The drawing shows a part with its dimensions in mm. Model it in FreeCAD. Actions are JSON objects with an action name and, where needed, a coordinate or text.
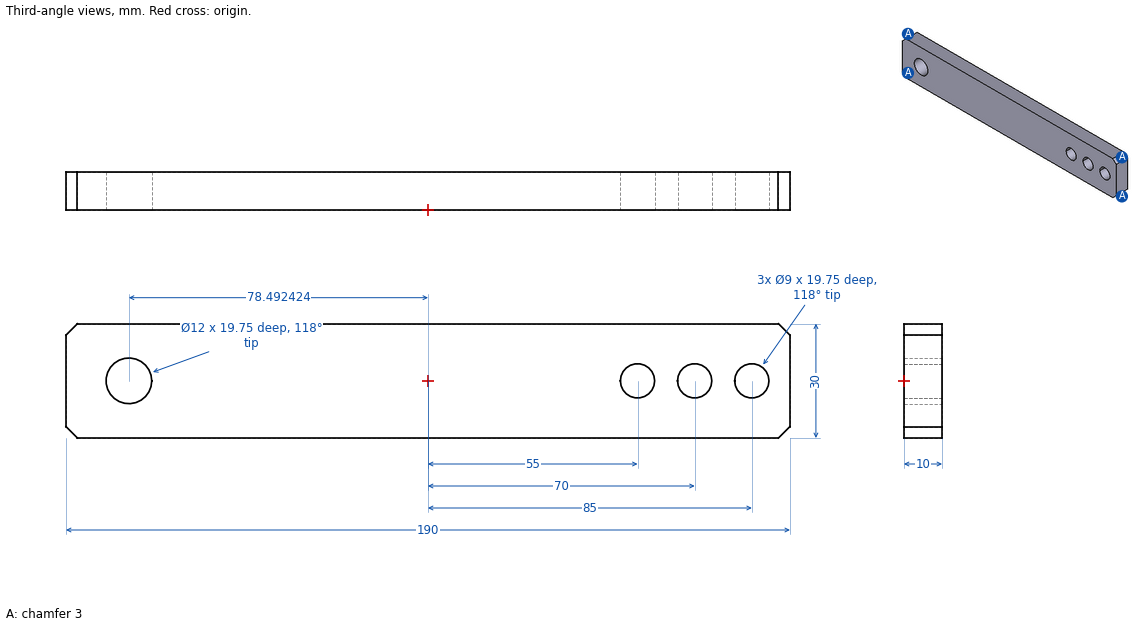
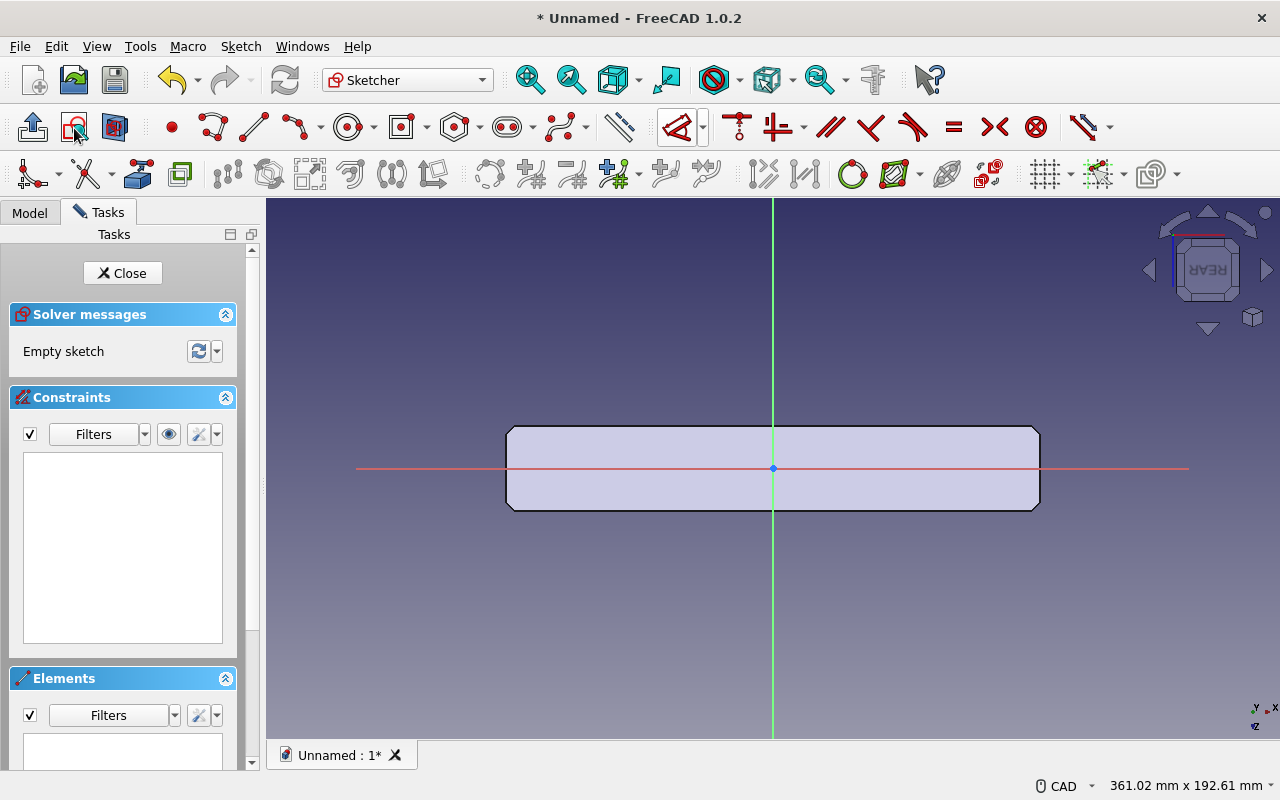
{"action": "scroll", "coordinate": [1057, 468], "scroll_direction": "up", "scroll_amount": 4}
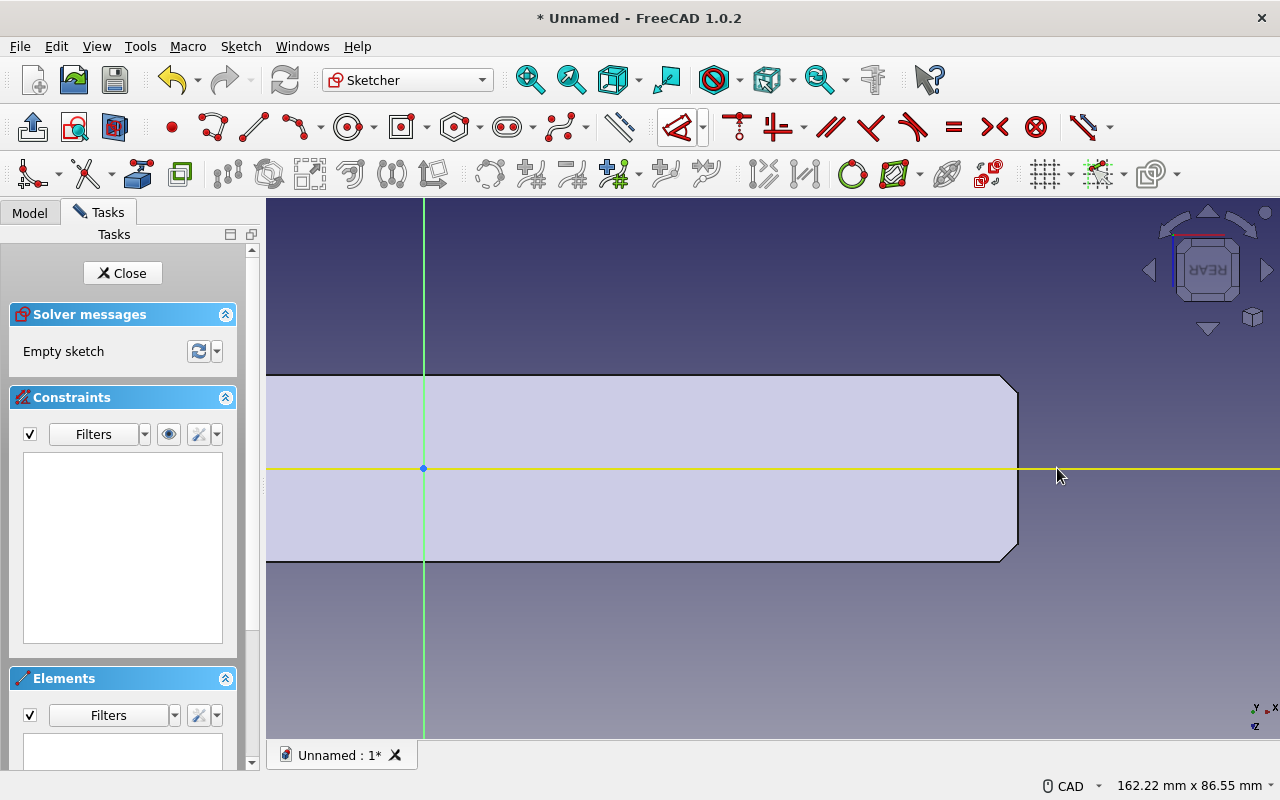
{"action": "left_click", "coordinate": [348, 128]}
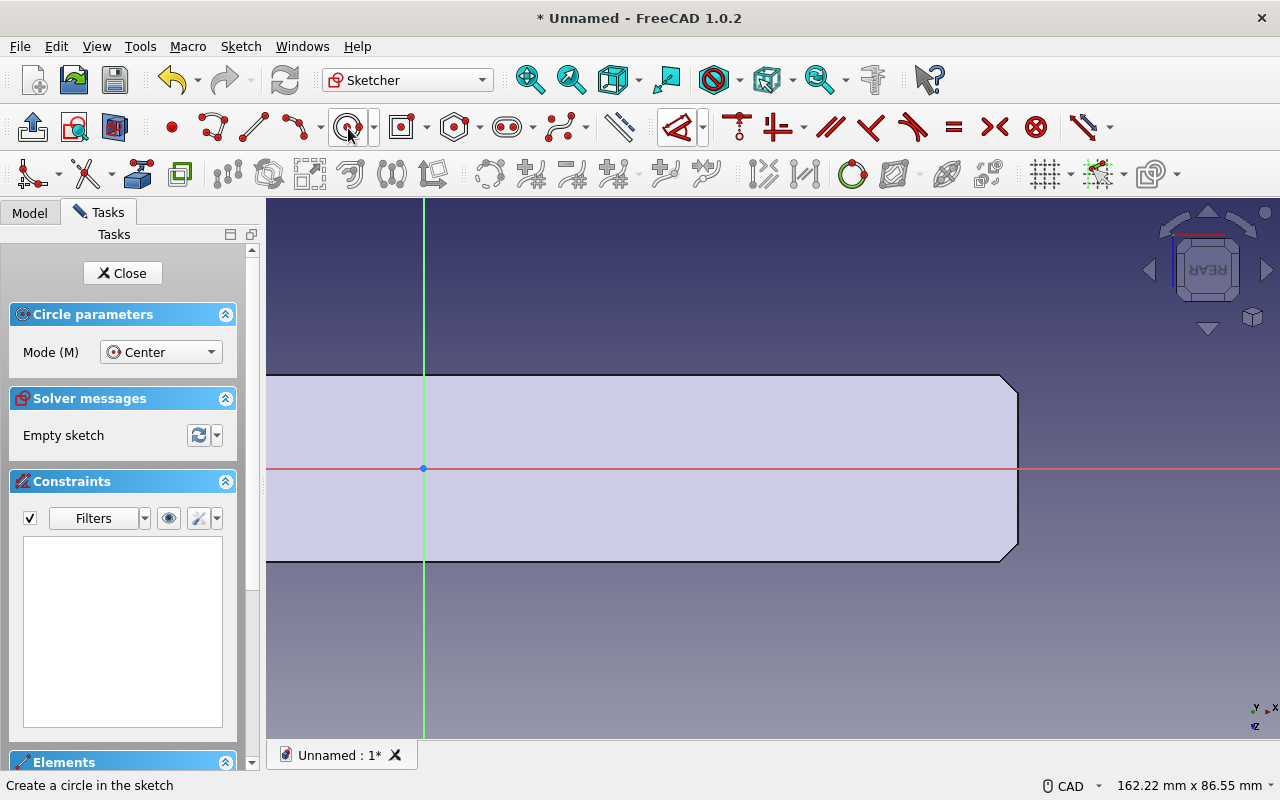
{"action": "left_click", "coordinate": [955, 468]}
{"action": "mouse_move", "coordinate": [975, 449]}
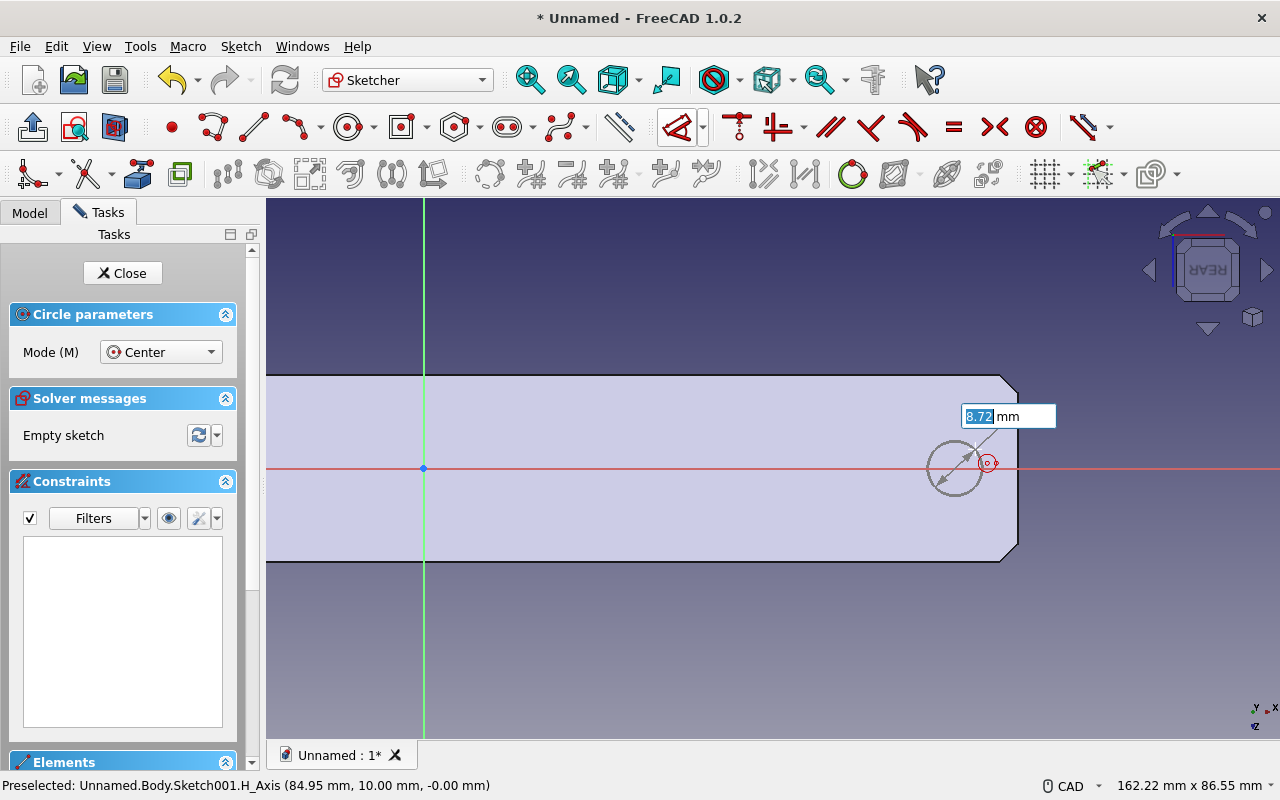
{"action": "type", "text": "9"}
{"action": "key", "text": "Return"}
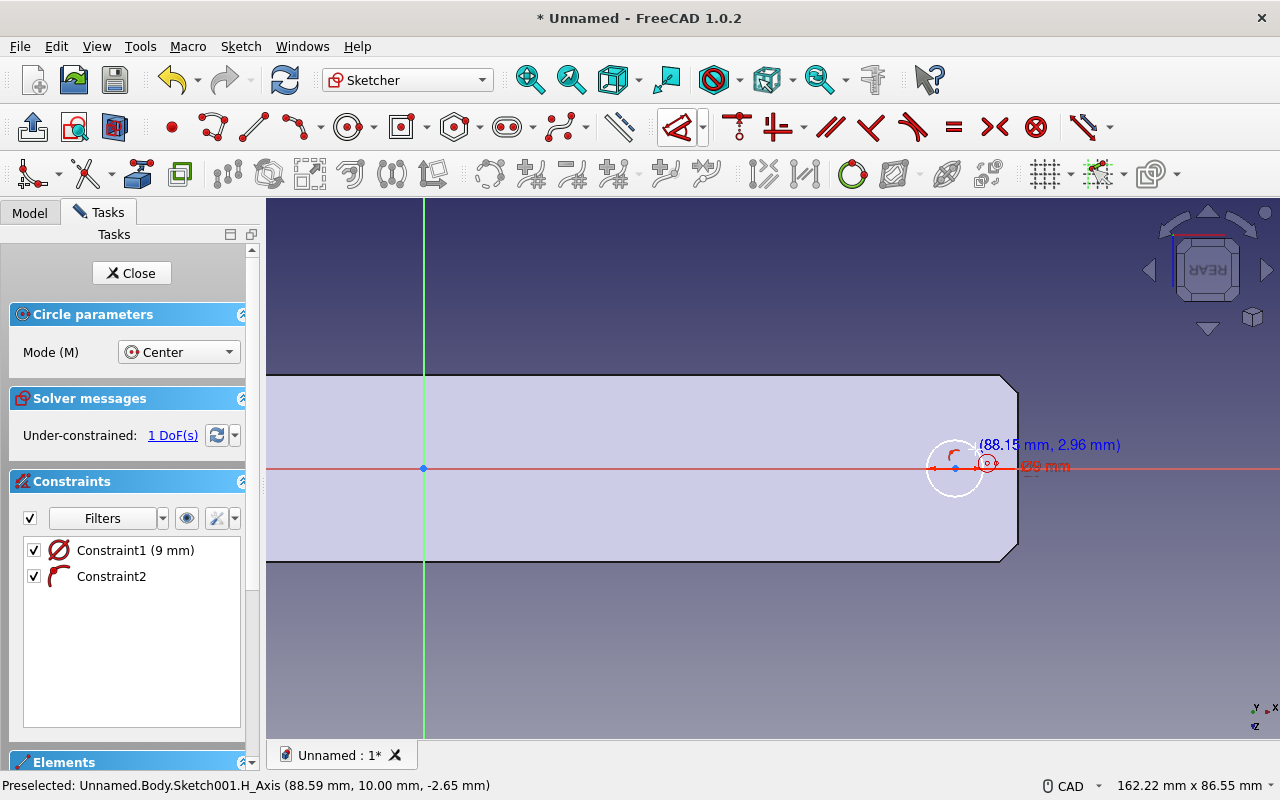
{"action": "left_click", "coordinate": [862, 468]}
{"action": "mouse_move", "coordinate": [881, 449]}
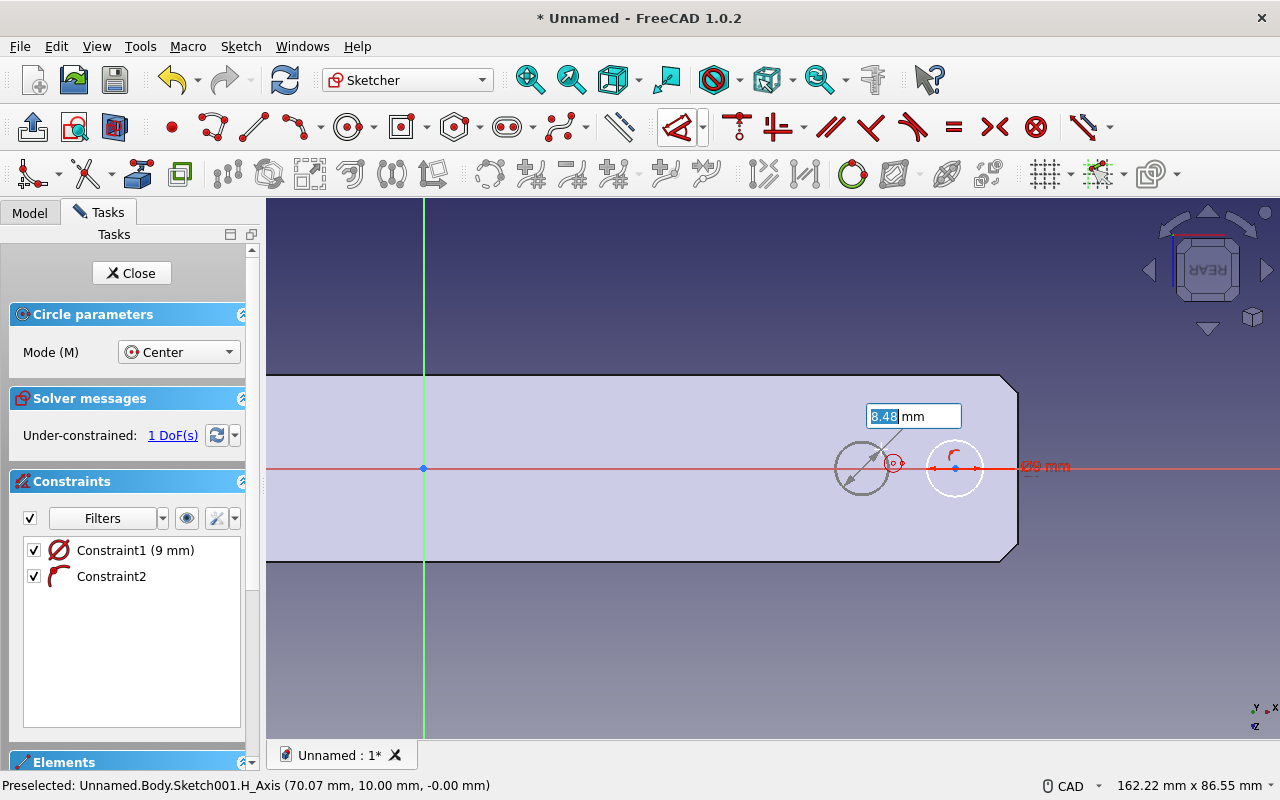
{"action": "type", "text": "9"}
{"action": "key", "text": "Return"}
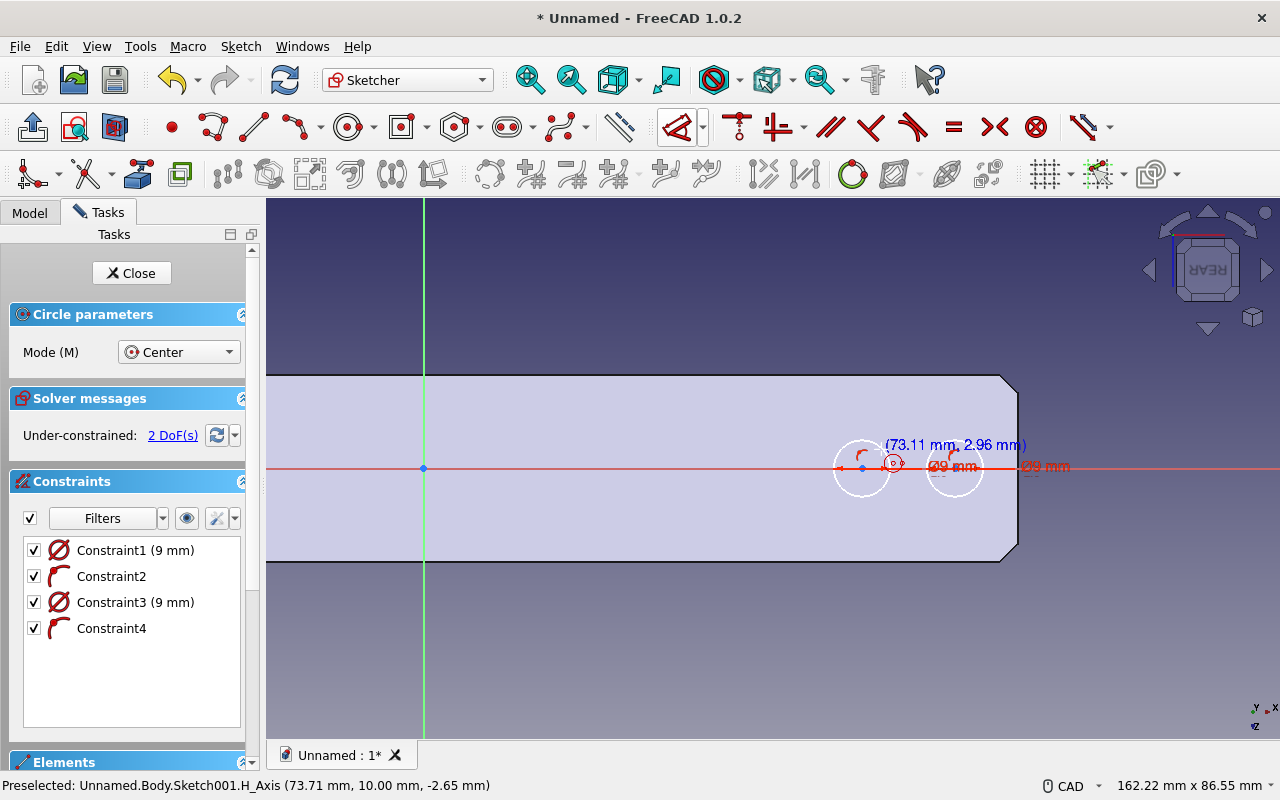
{"action": "left_click", "coordinate": [768, 468]}
{"action": "mouse_move", "coordinate": [788, 449]}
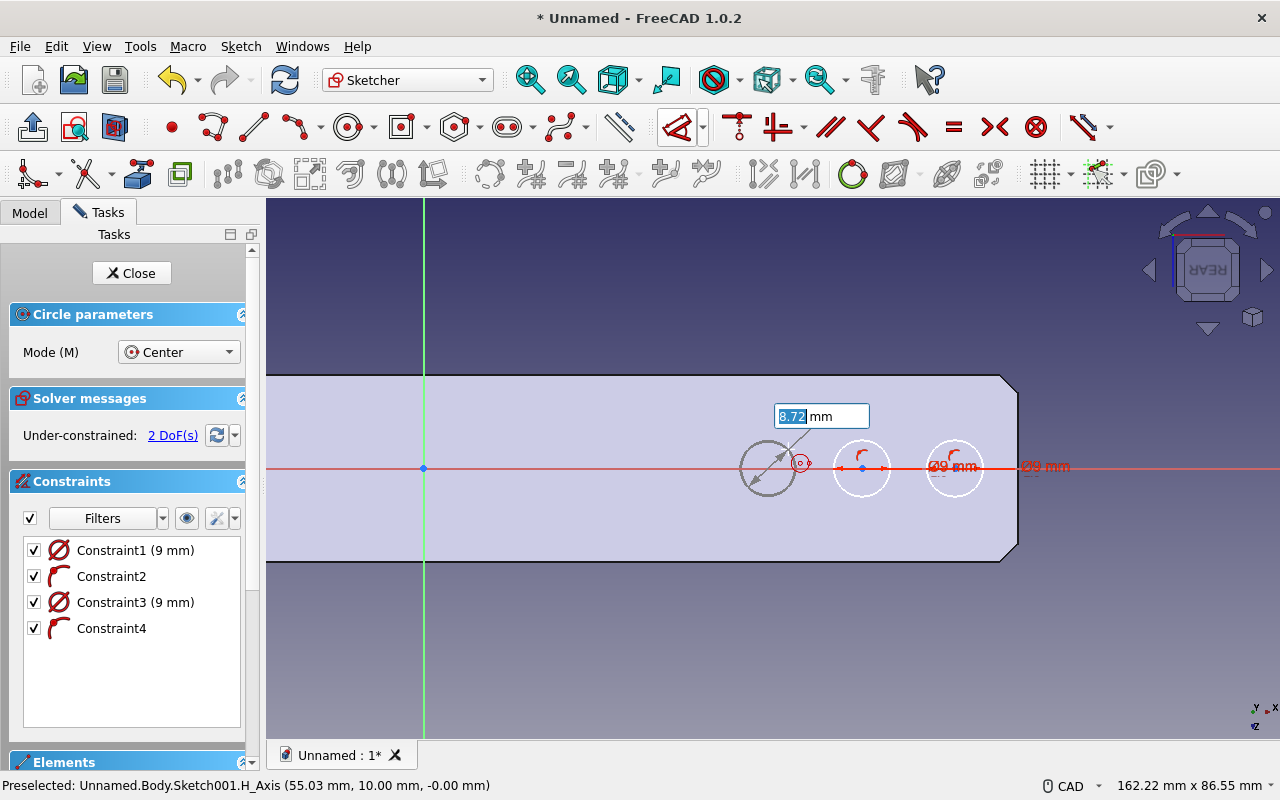
{"action": "type", "text": "9"}
{"action": "key", "text": "Return"}
{"action": "key", "text": "Escape"}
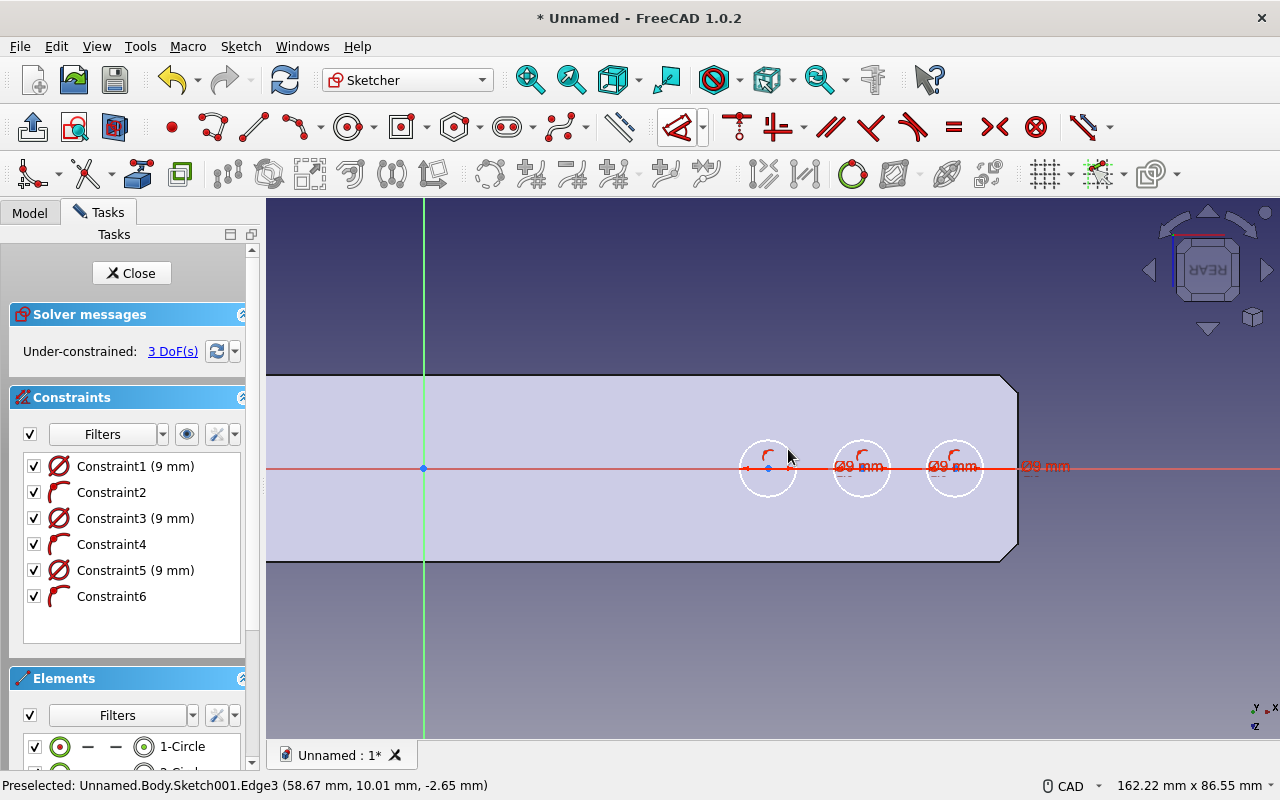
{"action": "key", "text": "d"}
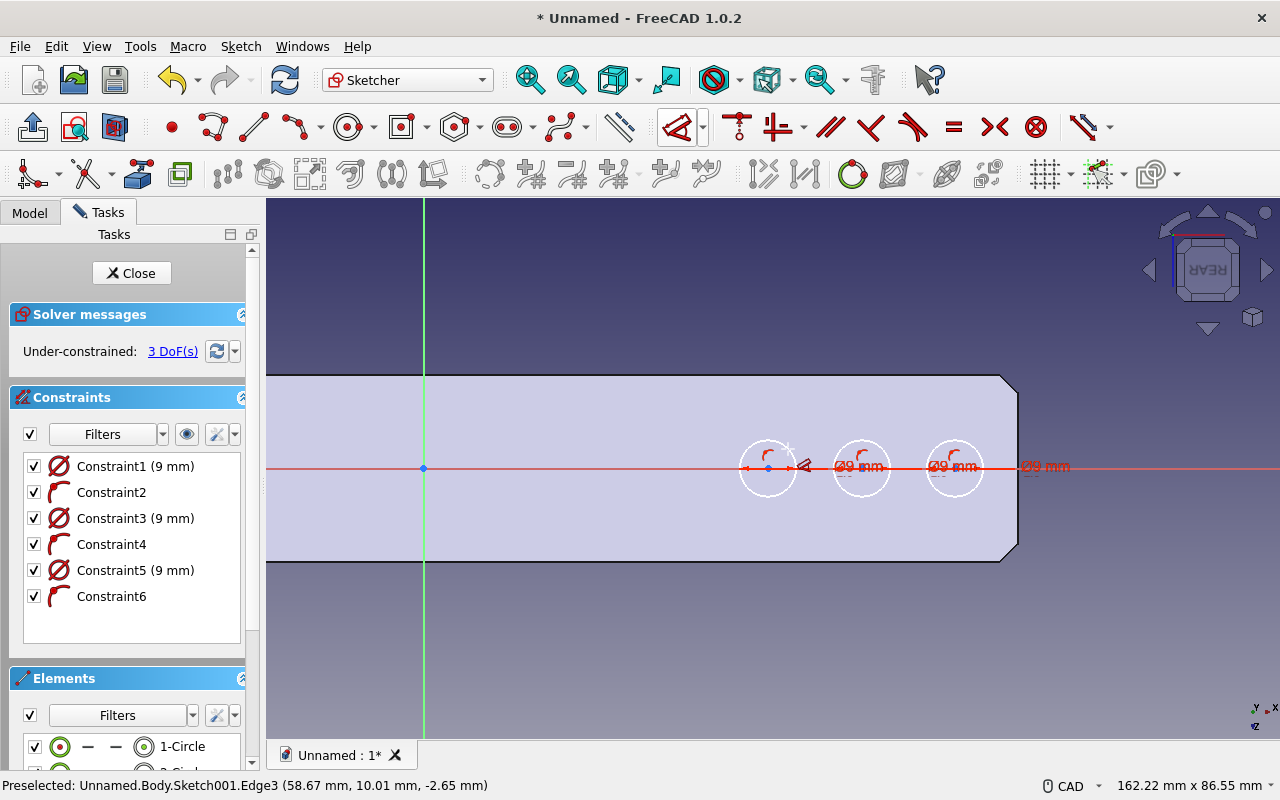
{"action": "left_click", "coordinate": [955, 468]}
{"action": "left_click", "coordinate": [689, 502]}